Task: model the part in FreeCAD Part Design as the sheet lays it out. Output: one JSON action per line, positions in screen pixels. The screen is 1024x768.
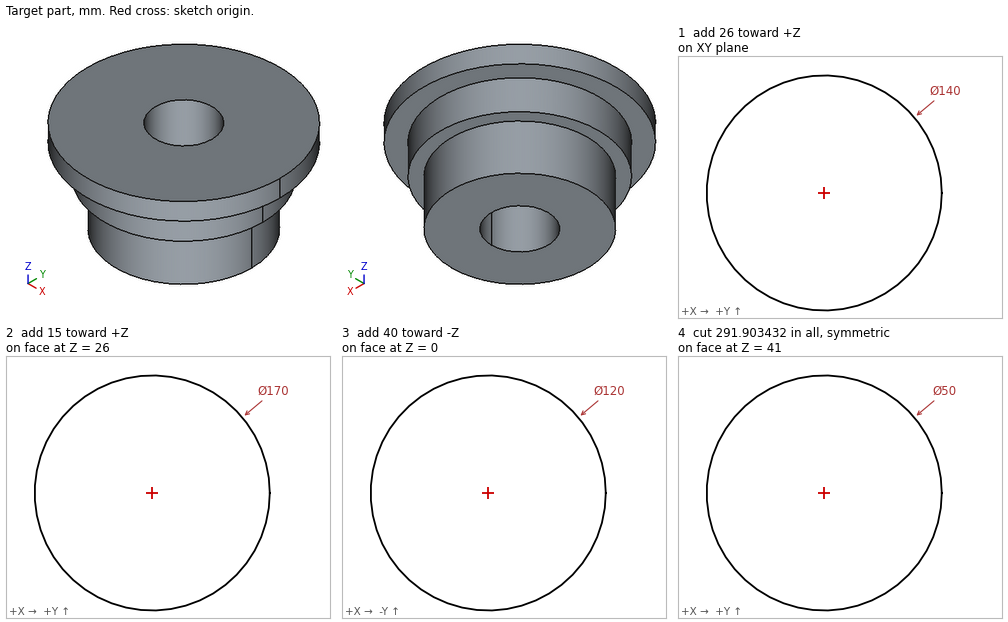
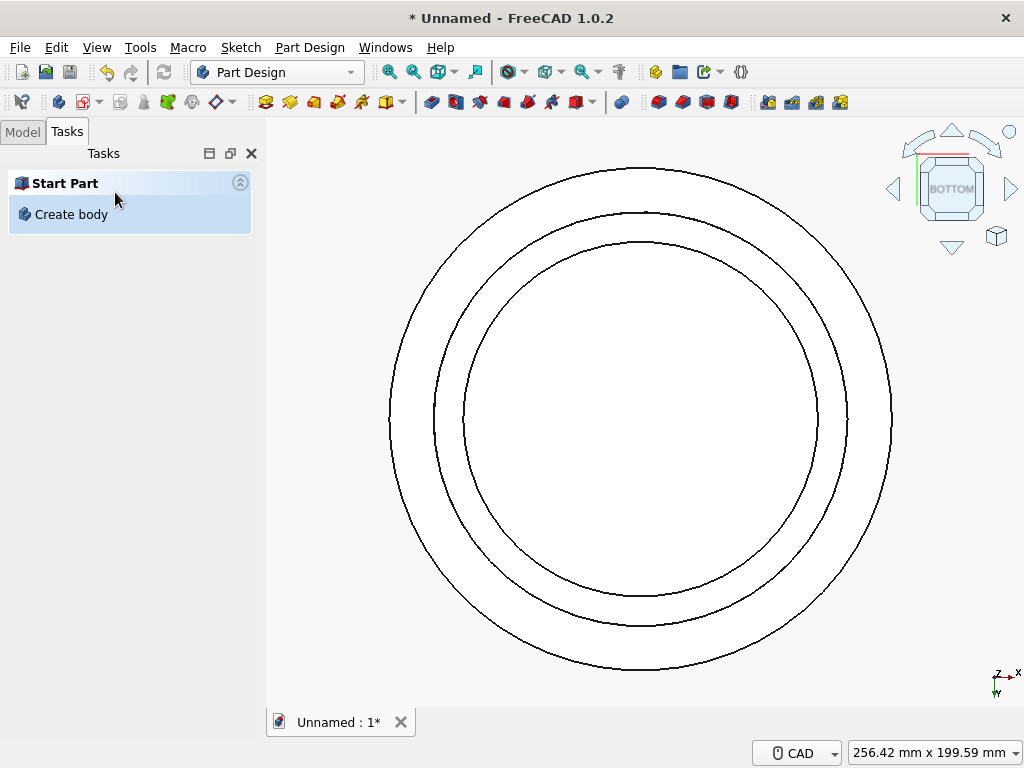
{"action": "key", "text": "0"}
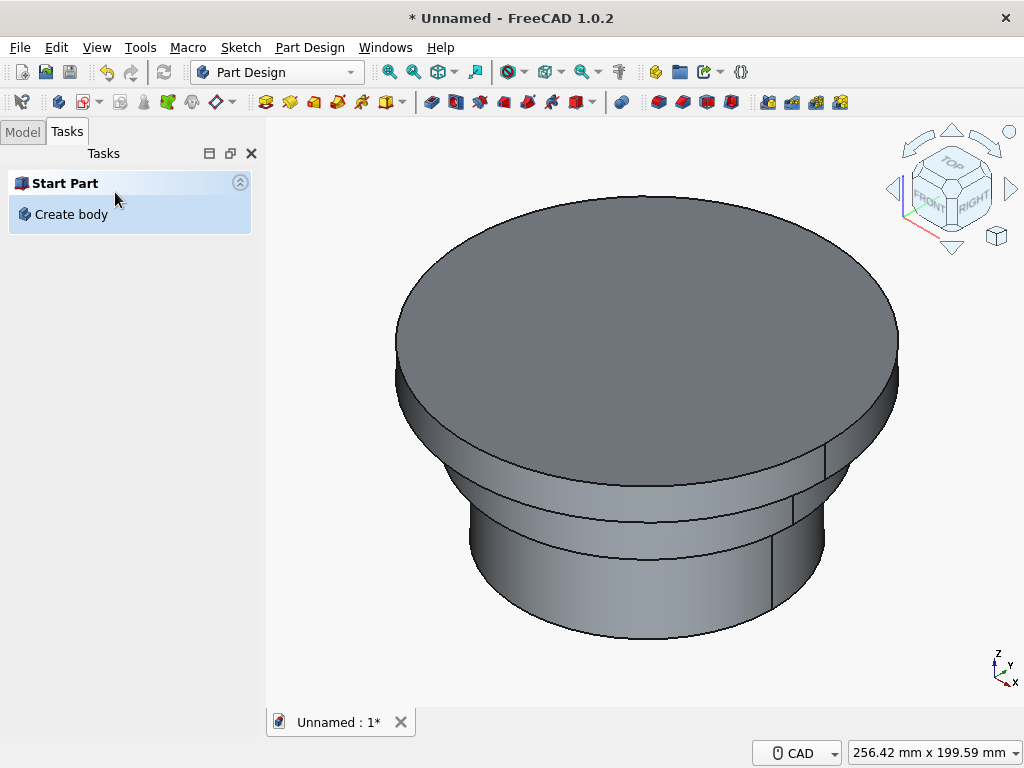
{"action": "key", "text": "v f"}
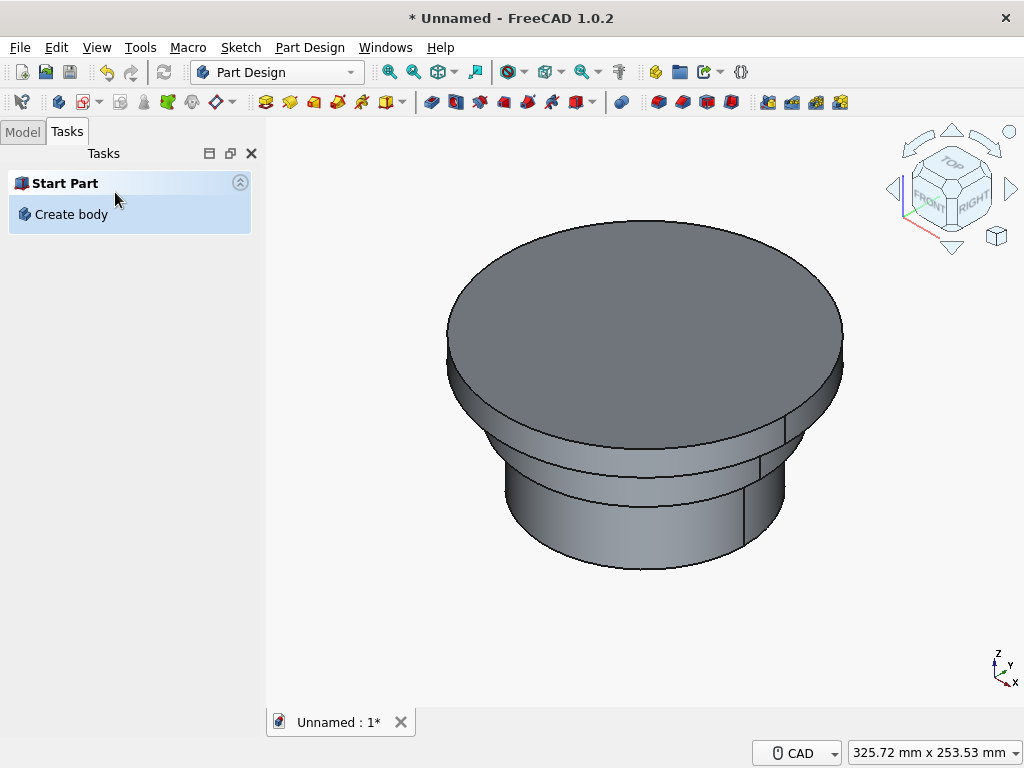
{"action": "left_click", "coordinate": [645, 334]}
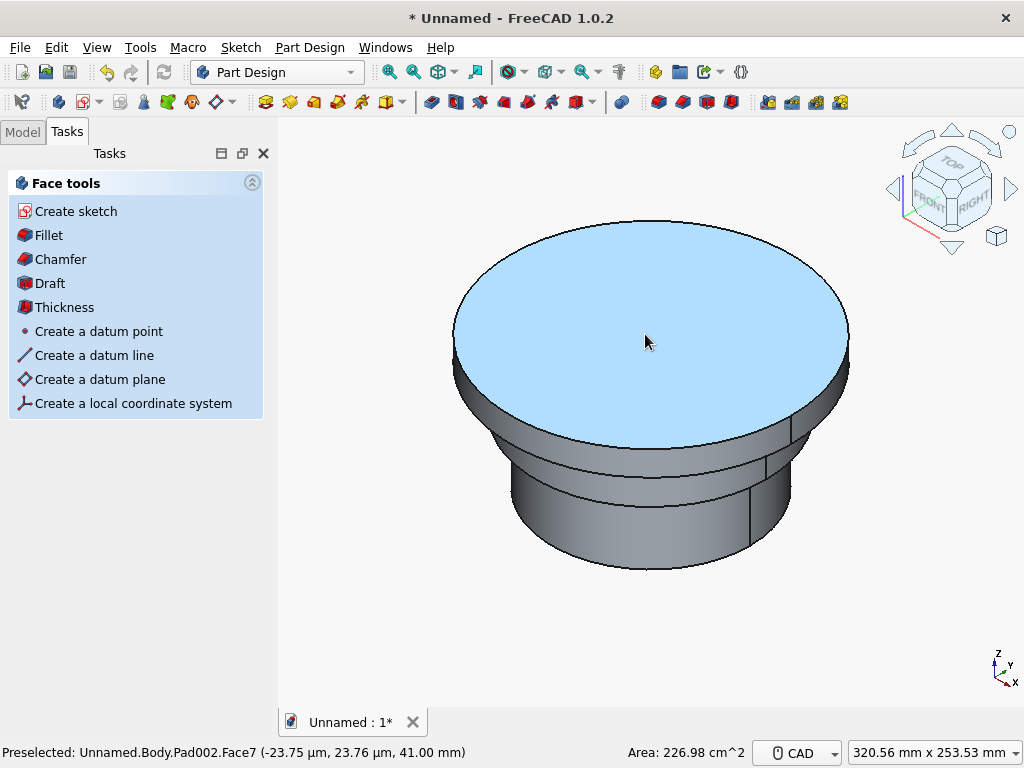
{"action": "left_click", "coordinate": [84, 102]}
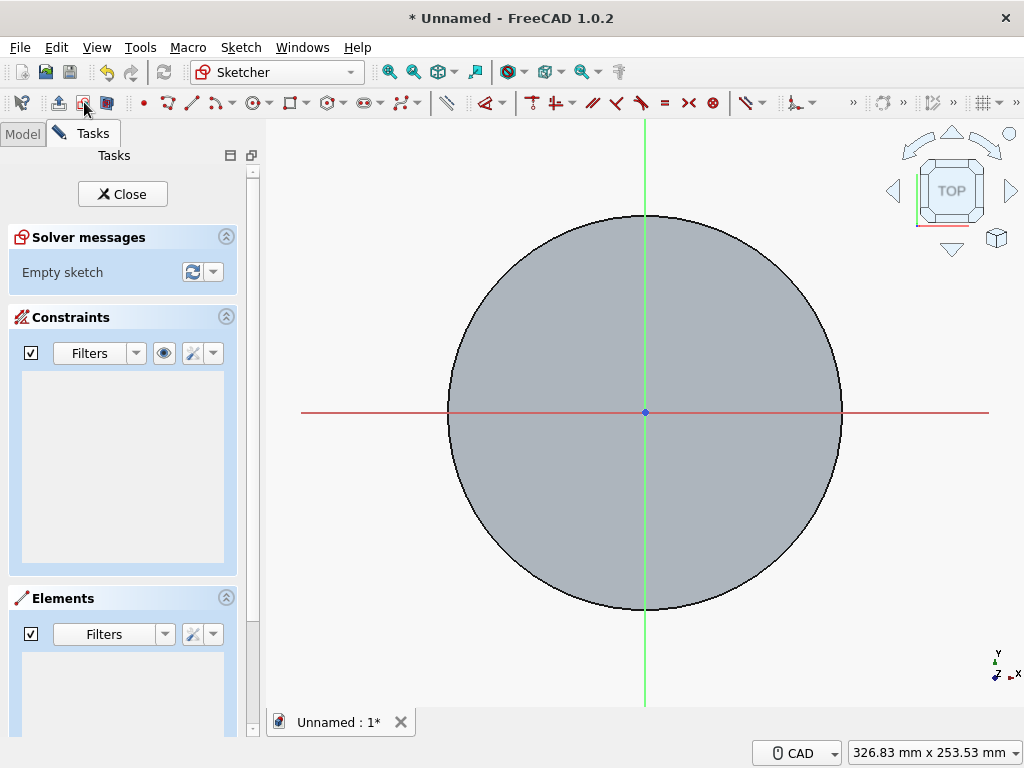
{"action": "scroll", "coordinate": [675, 413], "scroll_direction": "up", "scroll_amount": 6}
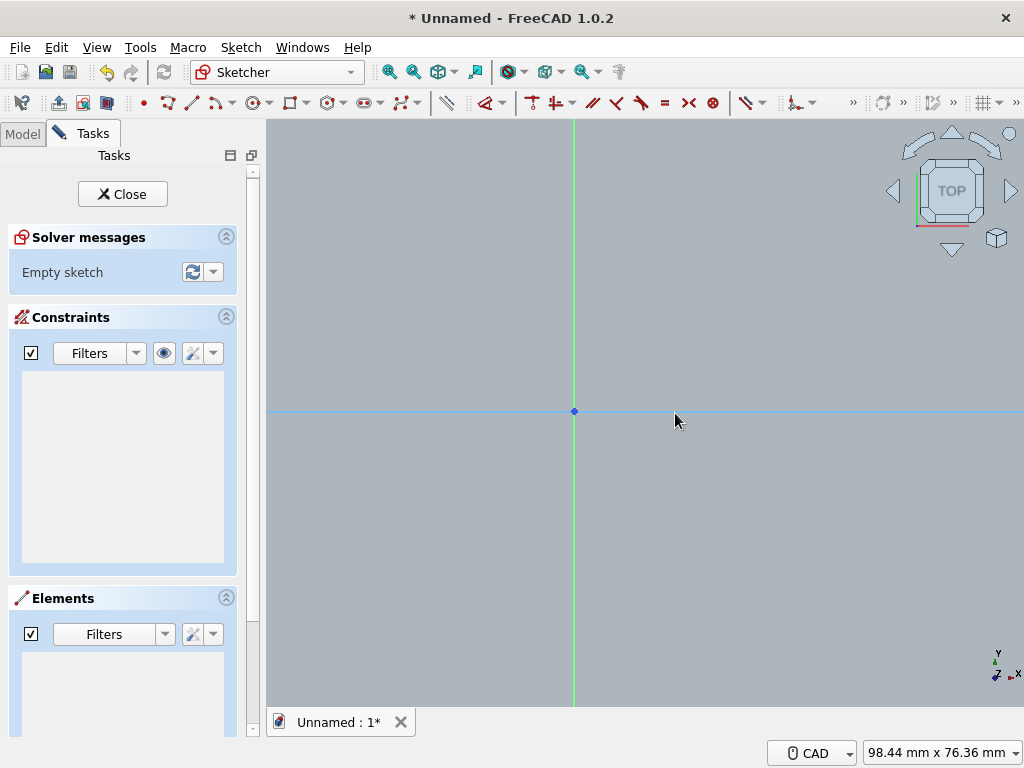
{"action": "left_click", "coordinate": [254, 104]}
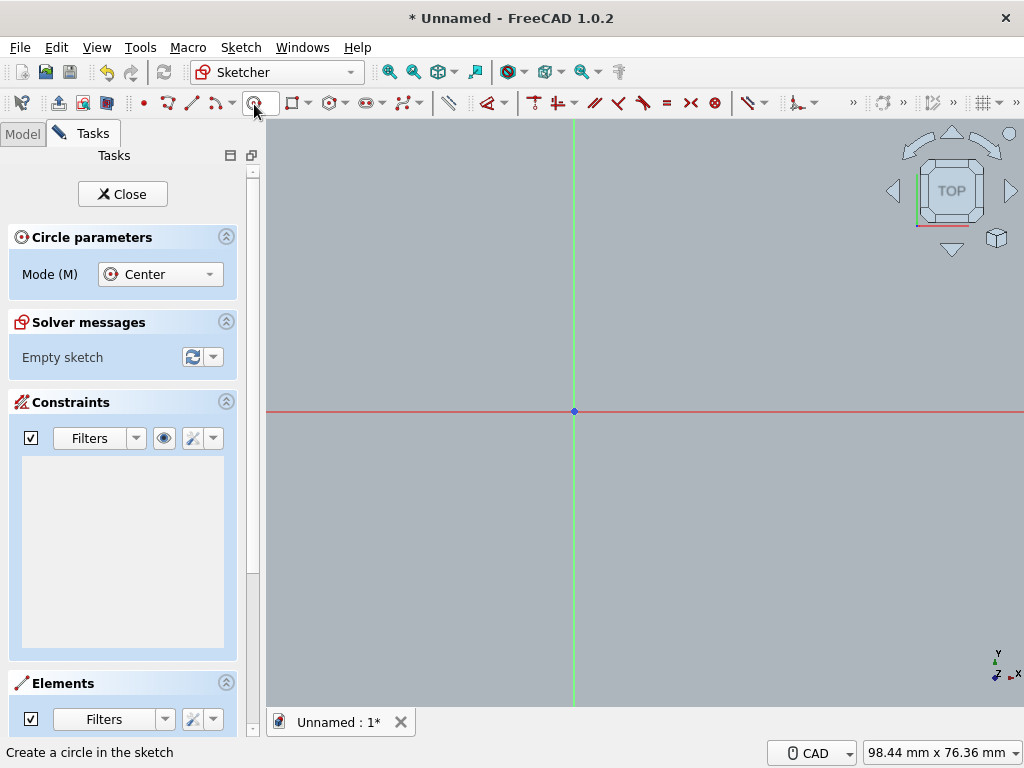
{"action": "left_click", "coordinate": [574, 412]}
{"action": "left_click", "coordinate": [710, 276]}
{"action": "key", "text": "Escape"}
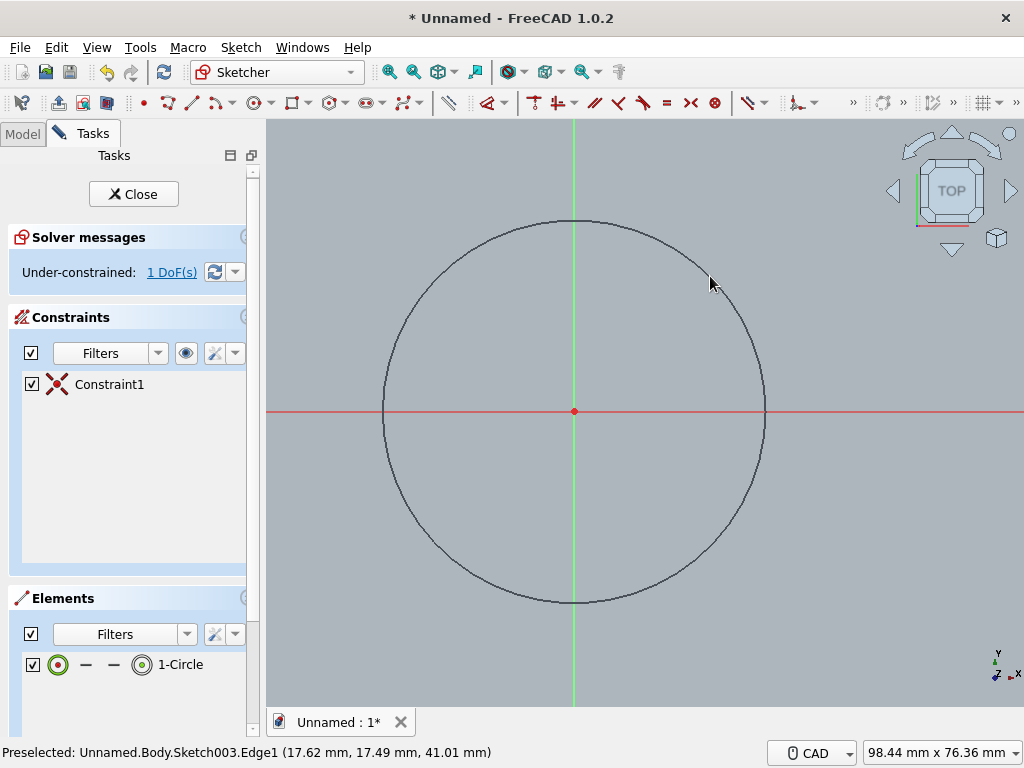
{"action": "key", "text": "d"}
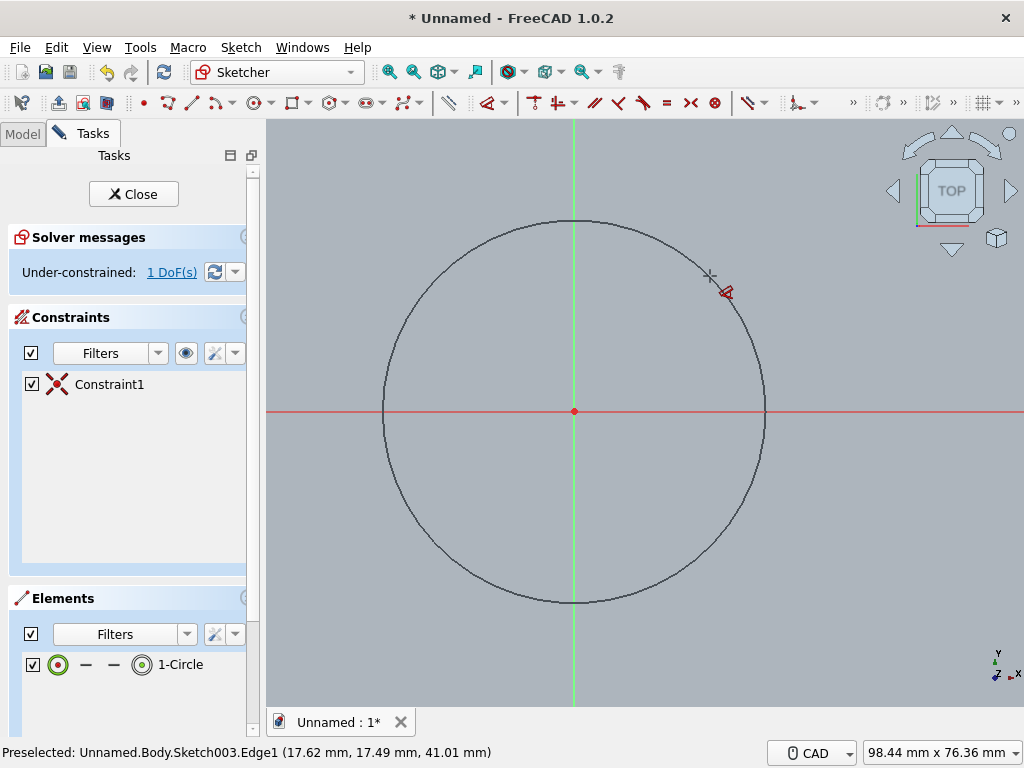
{"action": "left_click", "coordinate": [709, 276]}
{"action": "left_click", "coordinate": [732, 253]}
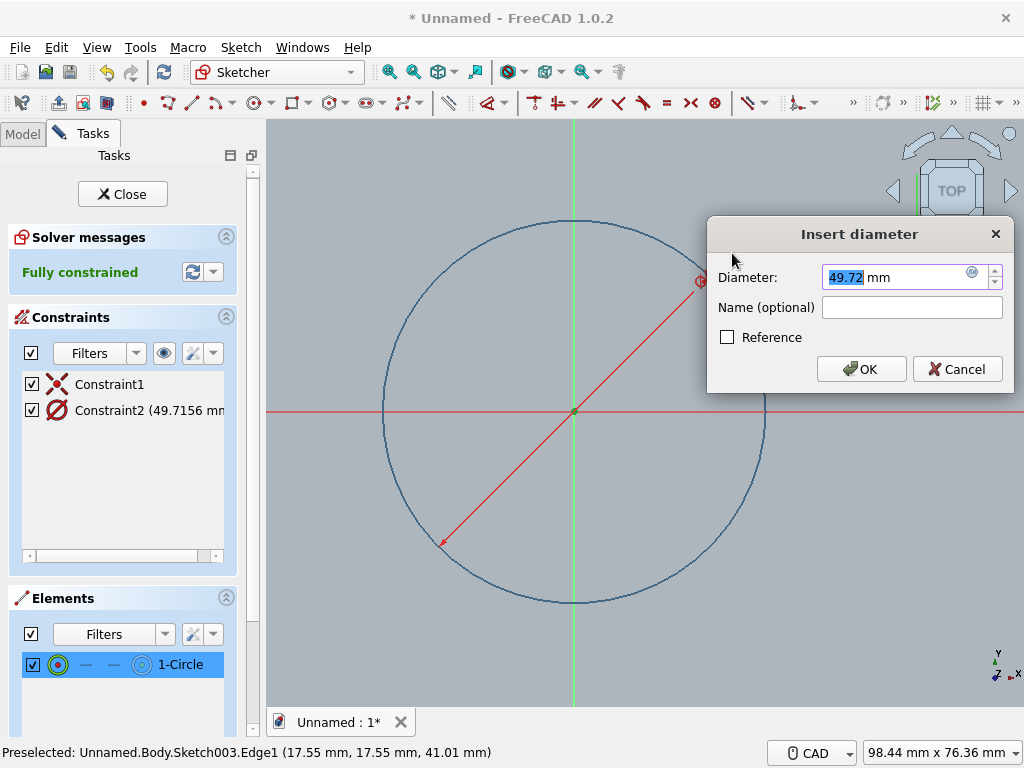
{"action": "type", "text": "50"}
{"action": "key", "text": "Return"}
{"action": "key", "text": "Escape"}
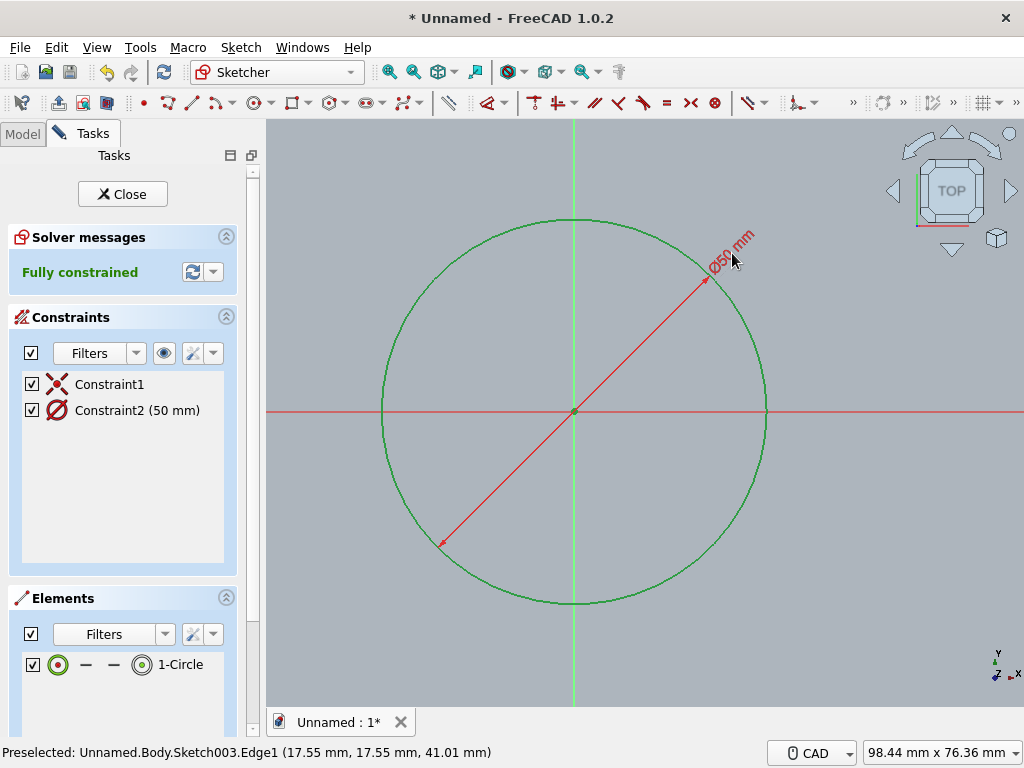
{"action": "left_click", "coordinate": [123, 194]}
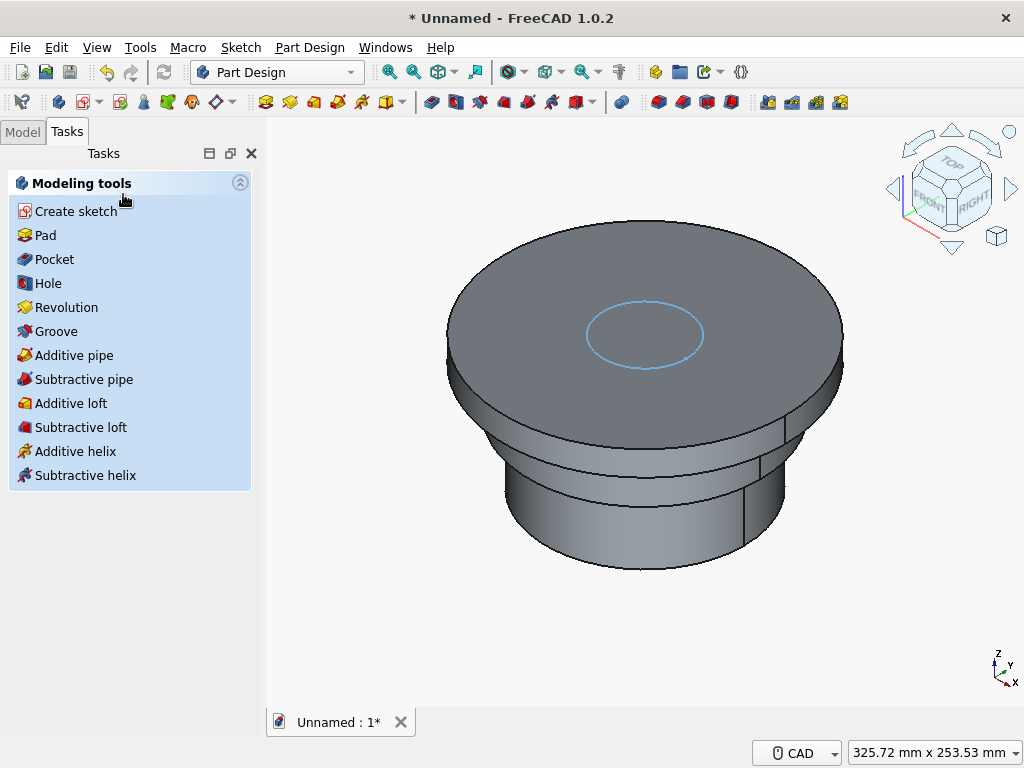
{"action": "left_click", "coordinate": [432, 102]}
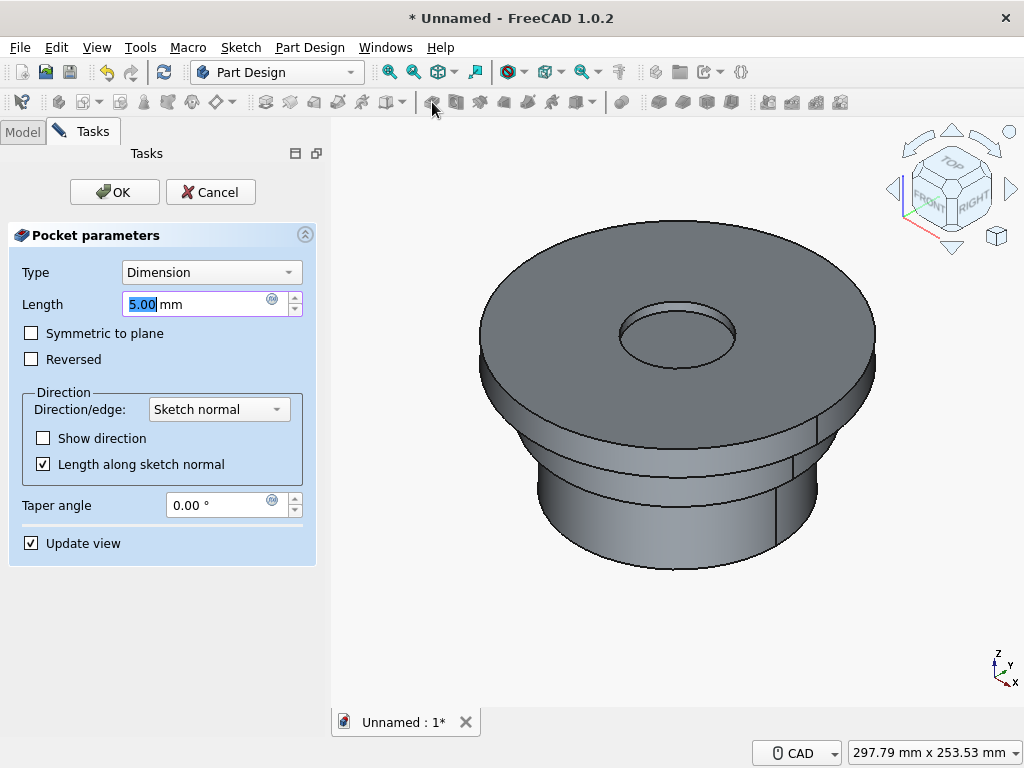
{"action": "type", "text": "291.903432"}
{"action": "key", "text": "Tab"}